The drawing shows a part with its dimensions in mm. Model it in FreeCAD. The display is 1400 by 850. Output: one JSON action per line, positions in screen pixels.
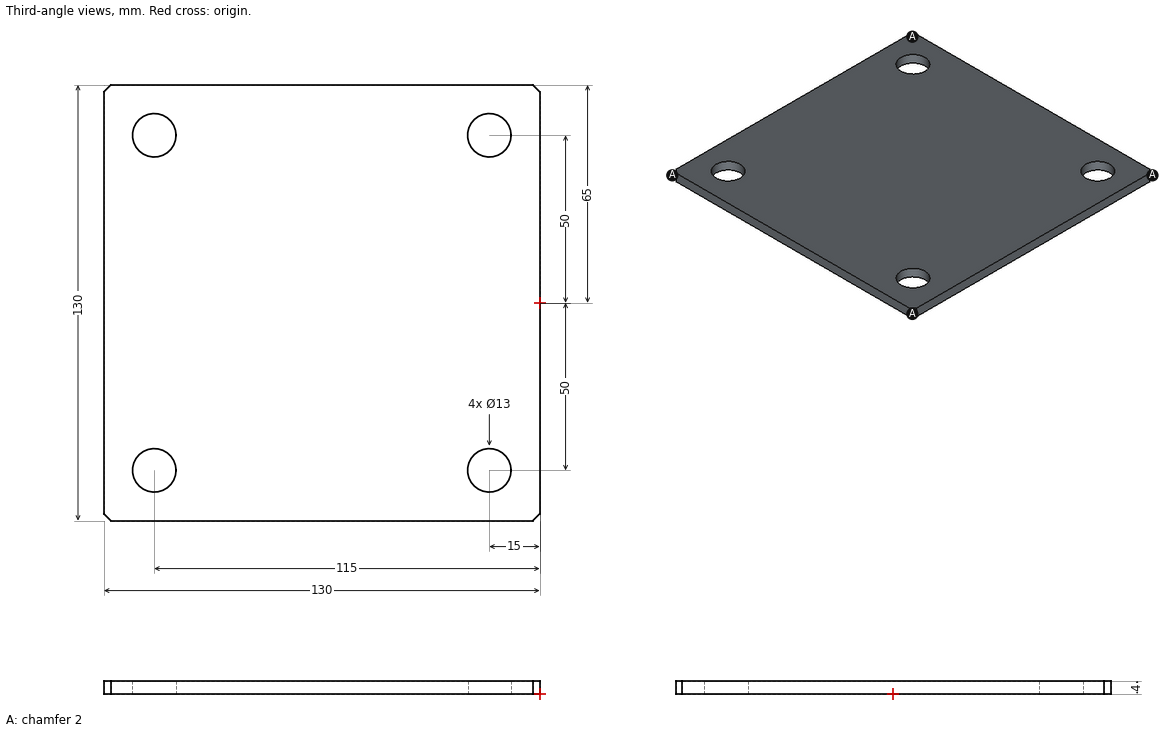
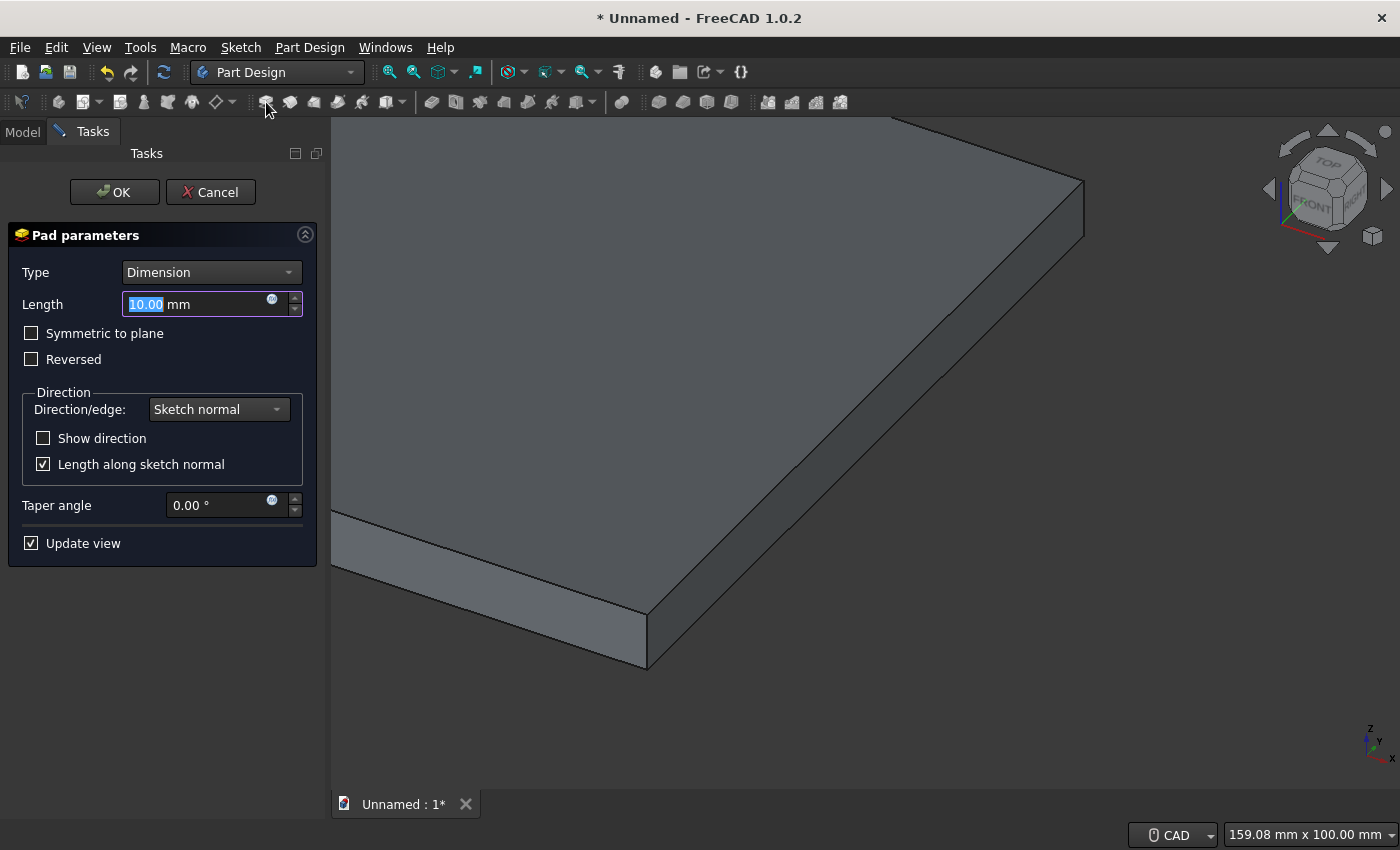
{"action": "type", "text": "4"}
{"action": "key", "text": "Tab"}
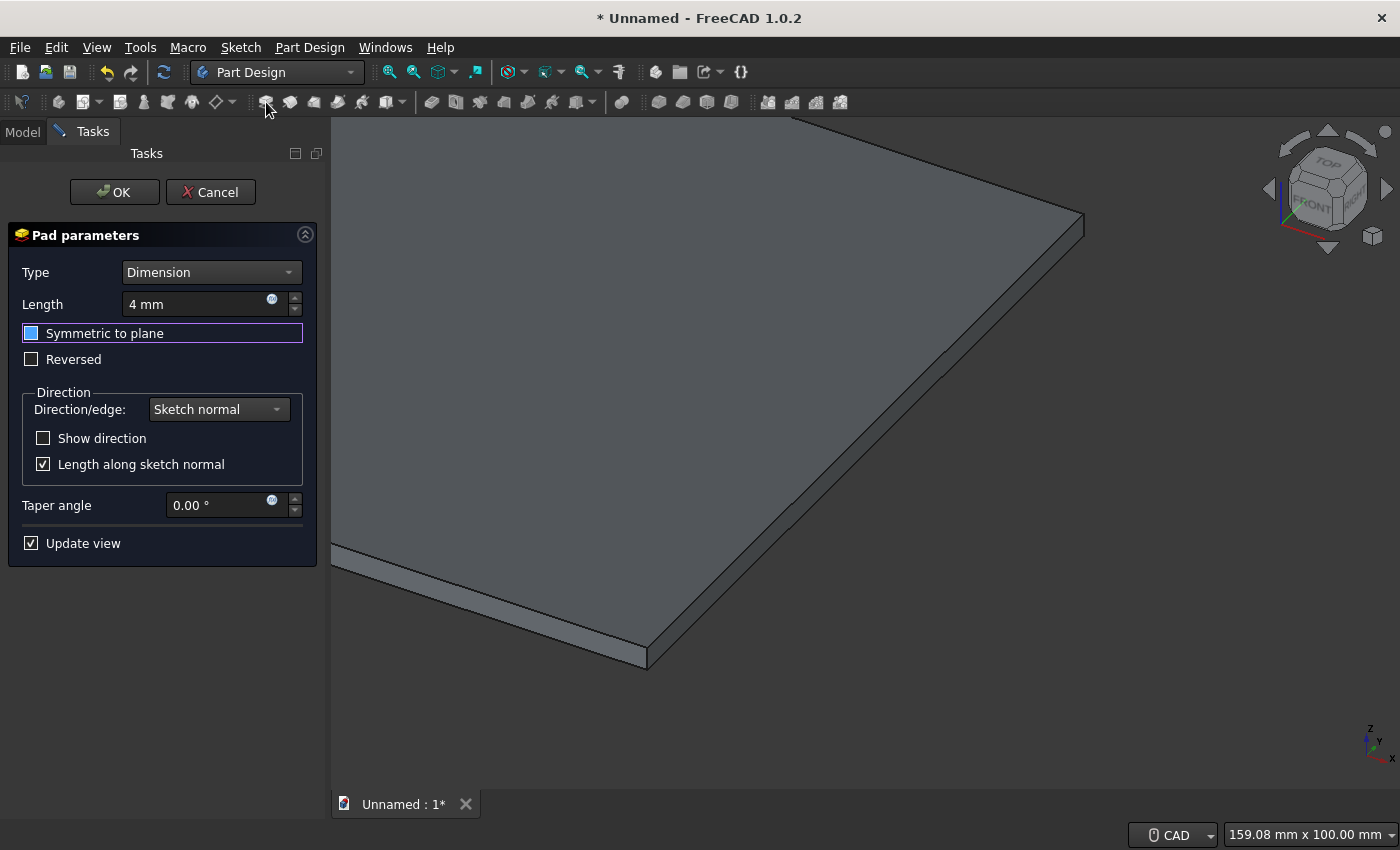
{"action": "left_click", "coordinate": [115, 192]}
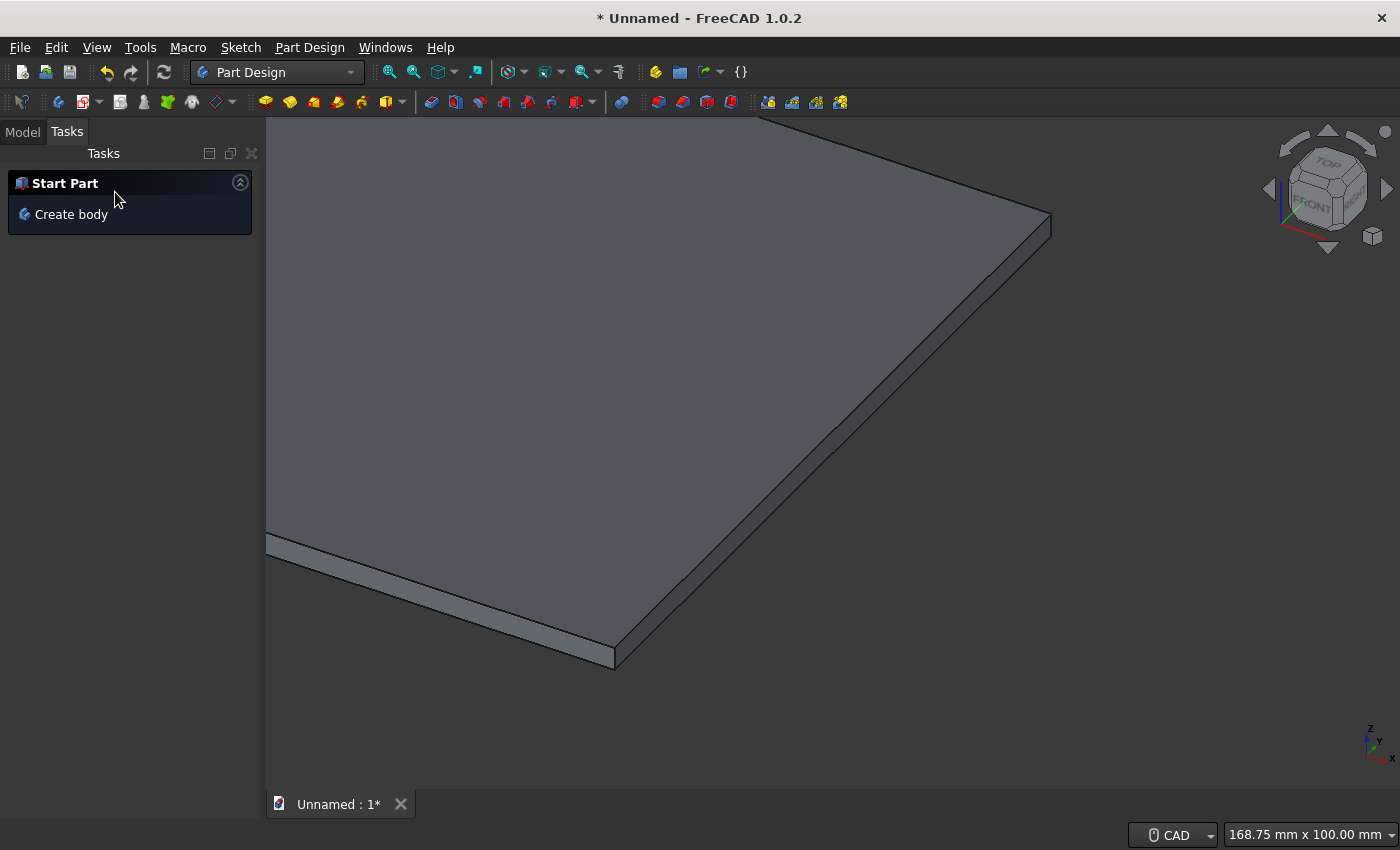
{"action": "left_click", "coordinate": [390, 72]}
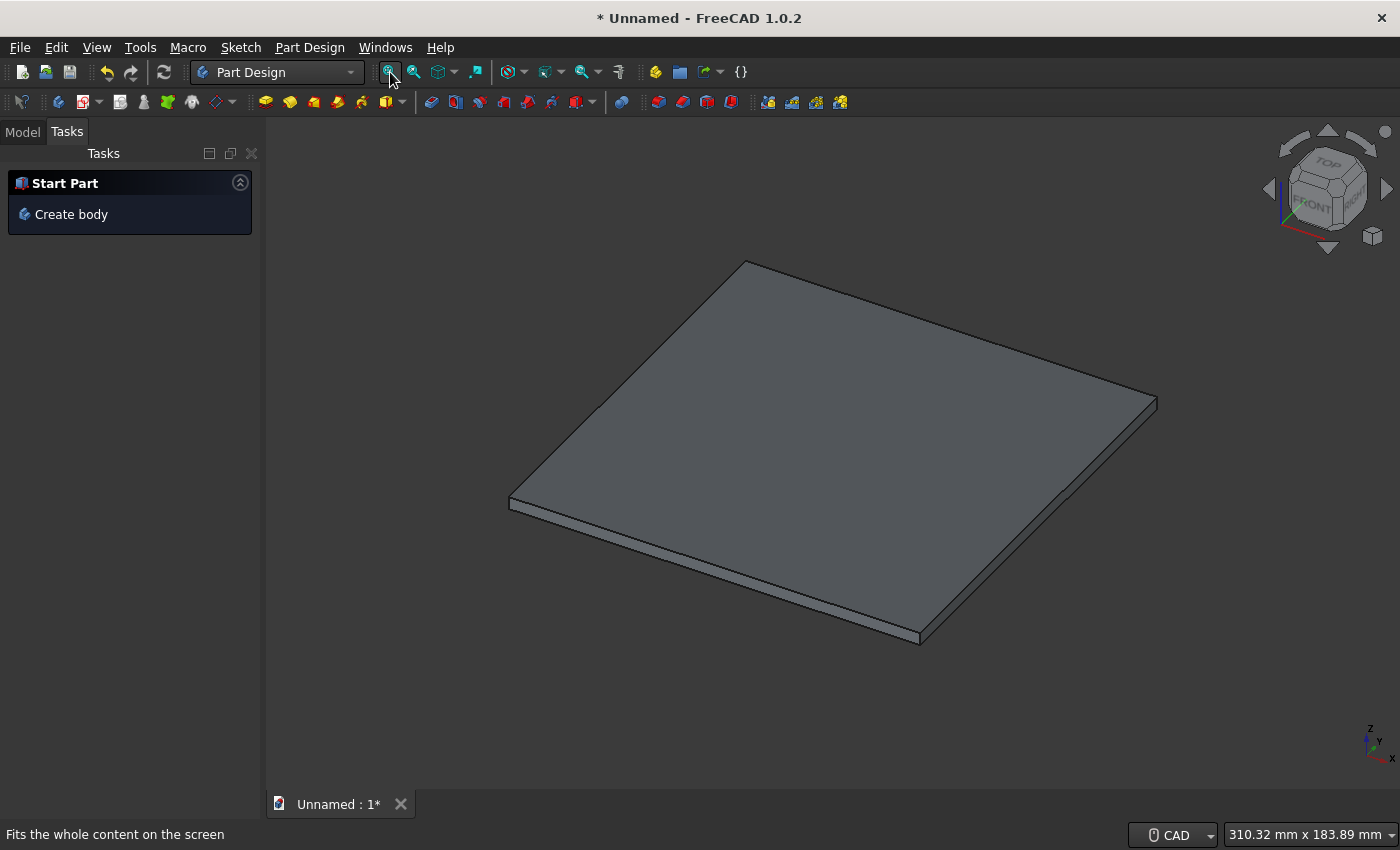
{"action": "left_click", "coordinate": [920, 639]}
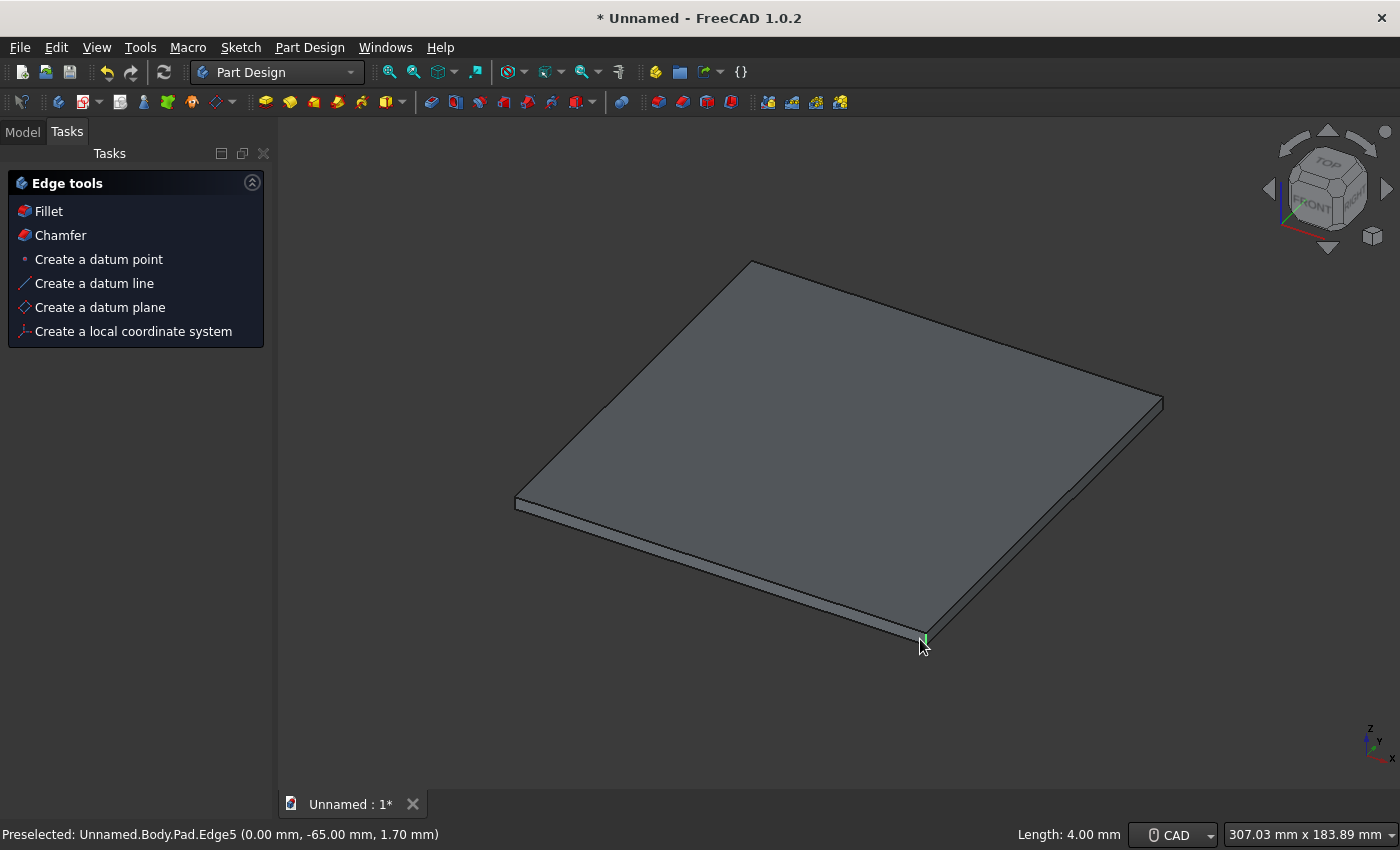
{"action": "scroll", "coordinate": [515, 502], "scroll_direction": "up", "scroll_amount": 6}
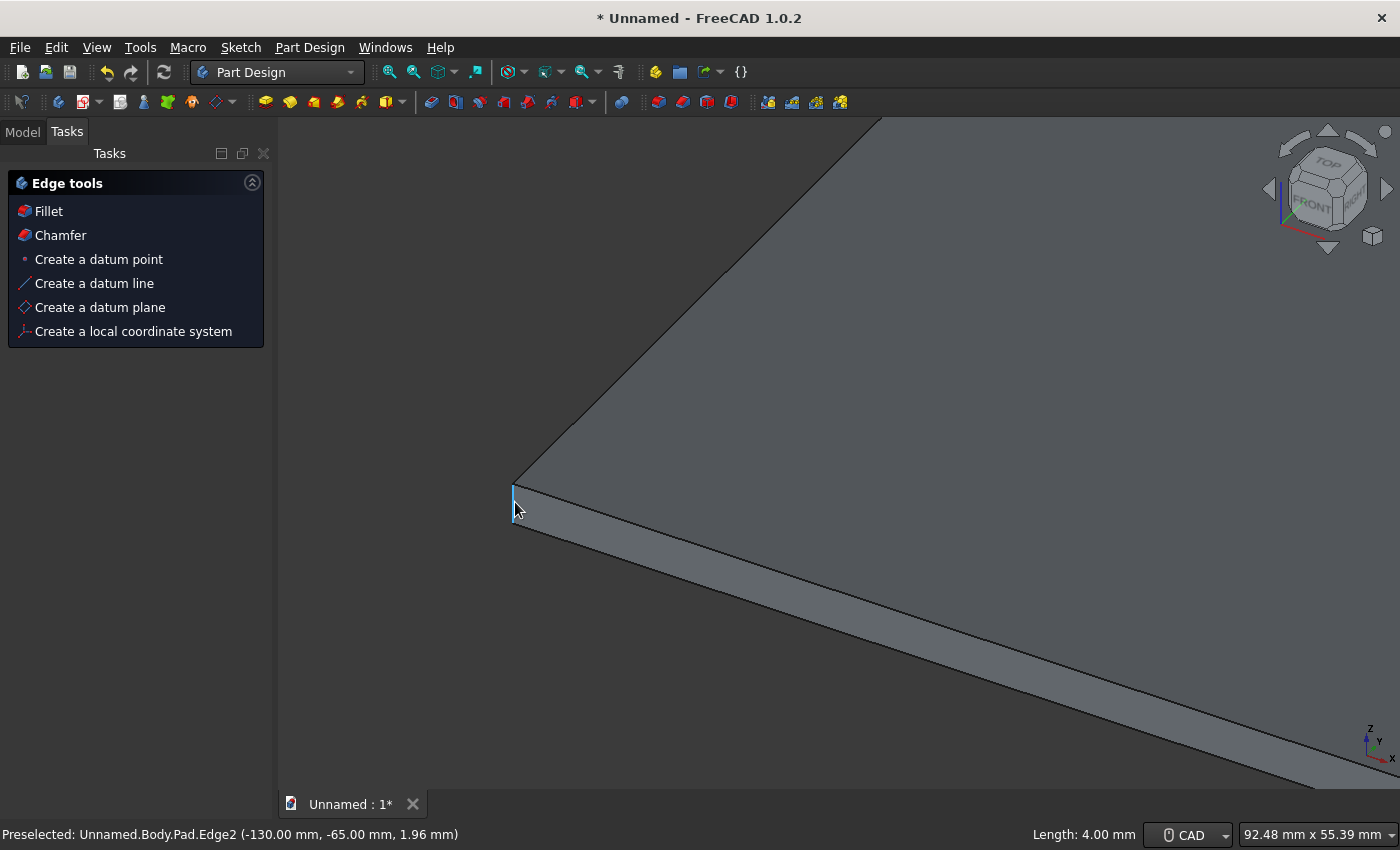
{"action": "left_click", "coordinate": [390, 72]}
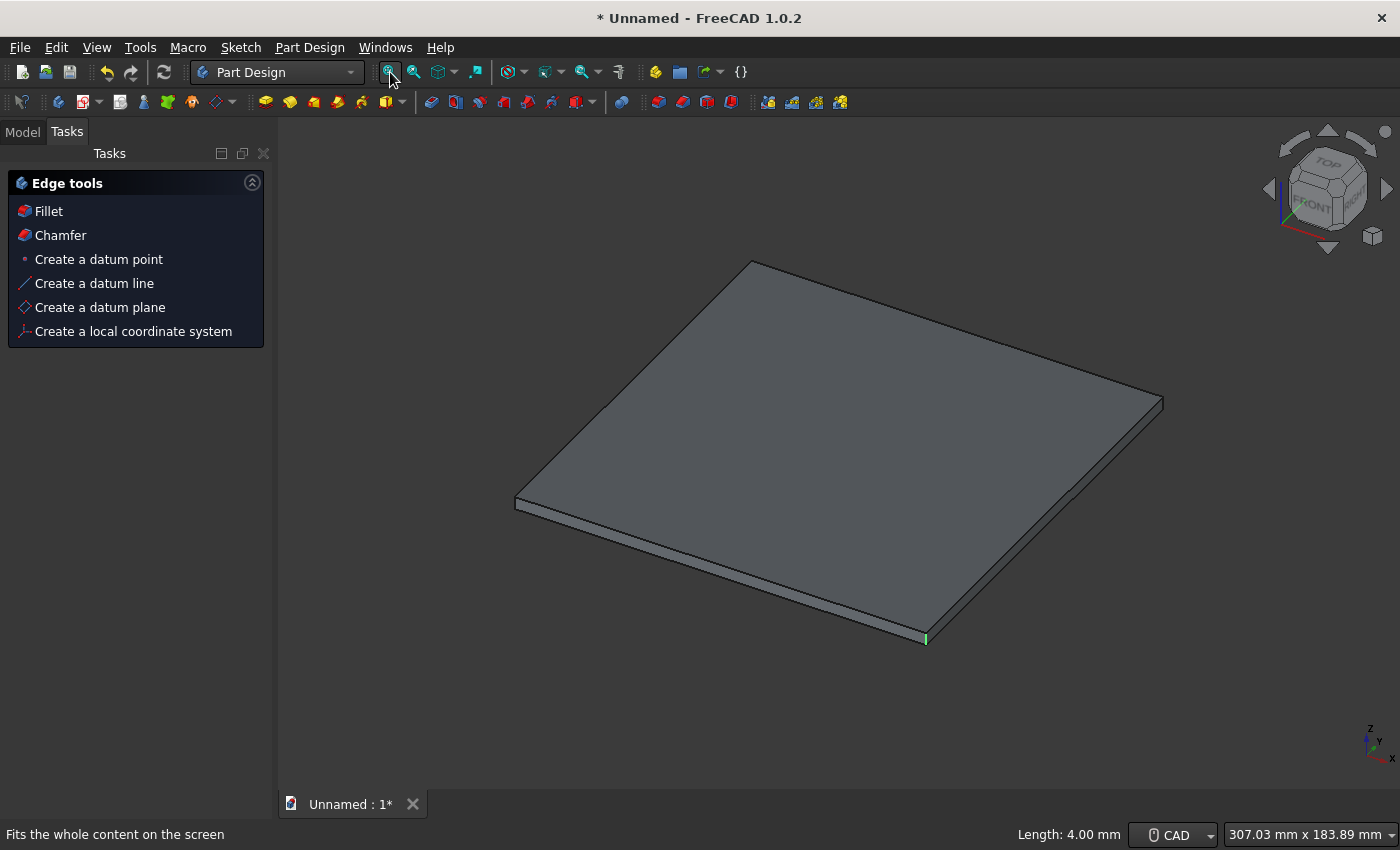
{"action": "key", "text": "0"}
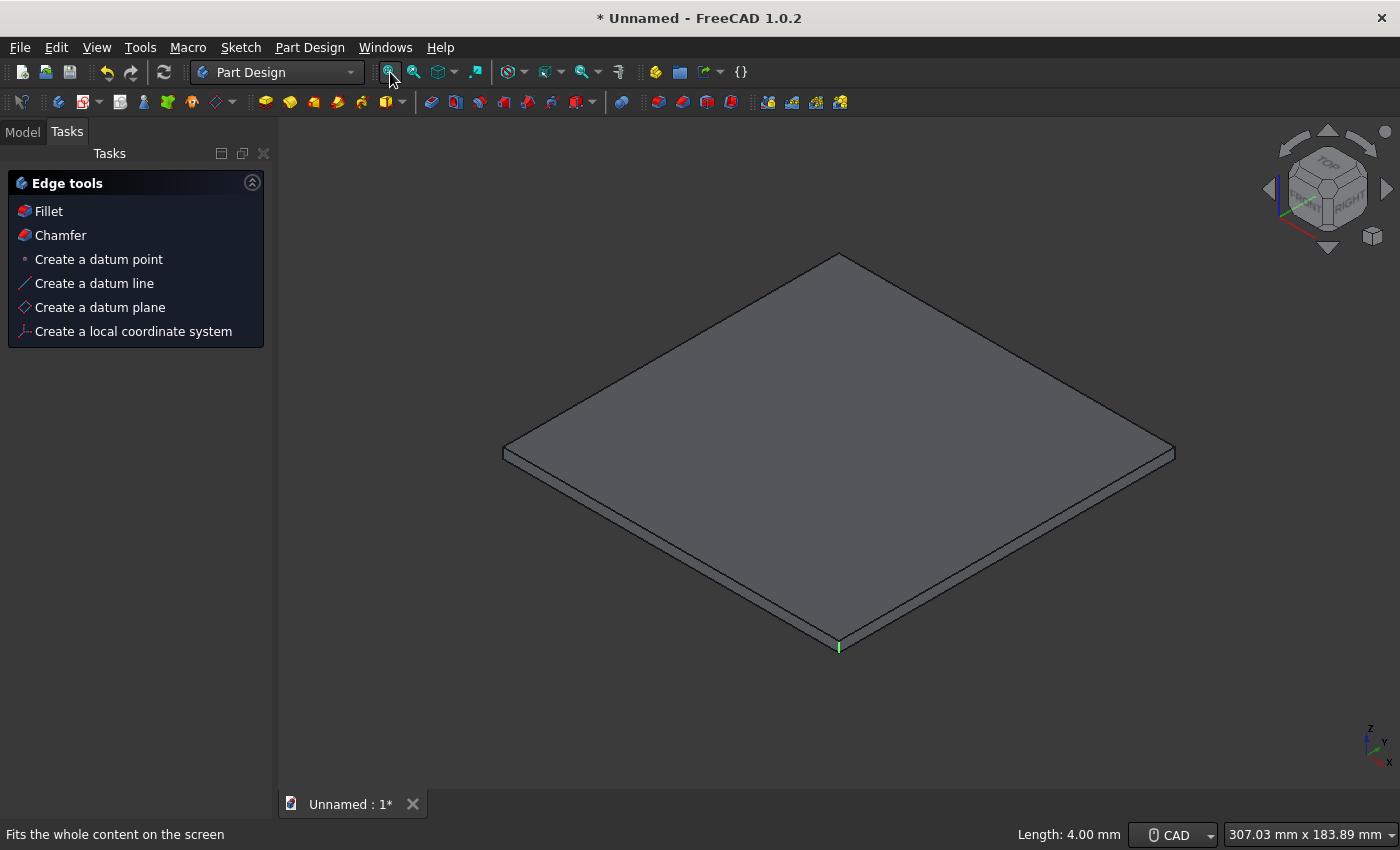
{"action": "scroll", "coordinate": [503, 452], "scroll_direction": "up", "scroll_amount": 6}